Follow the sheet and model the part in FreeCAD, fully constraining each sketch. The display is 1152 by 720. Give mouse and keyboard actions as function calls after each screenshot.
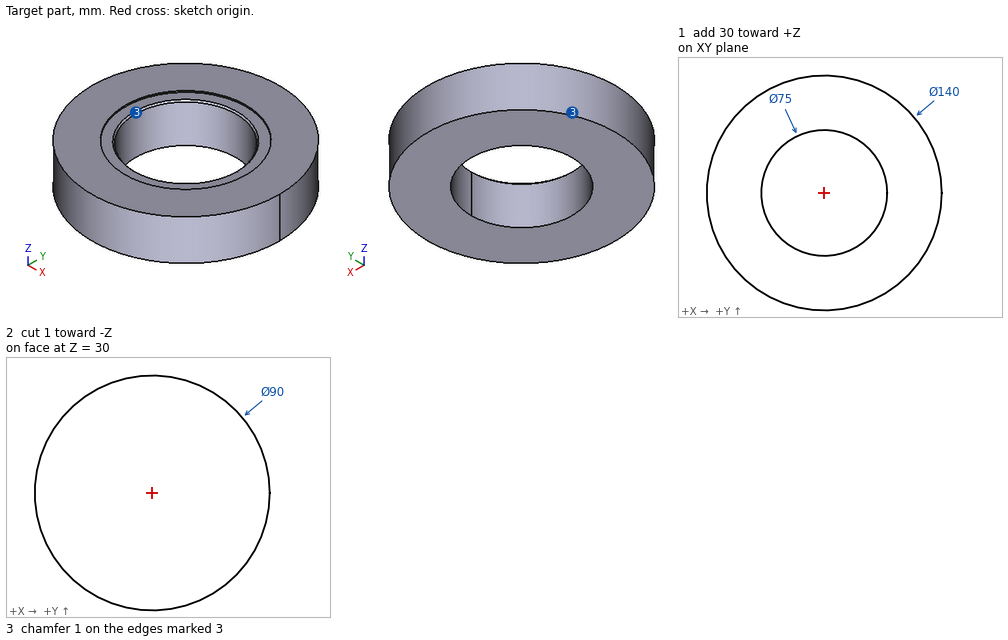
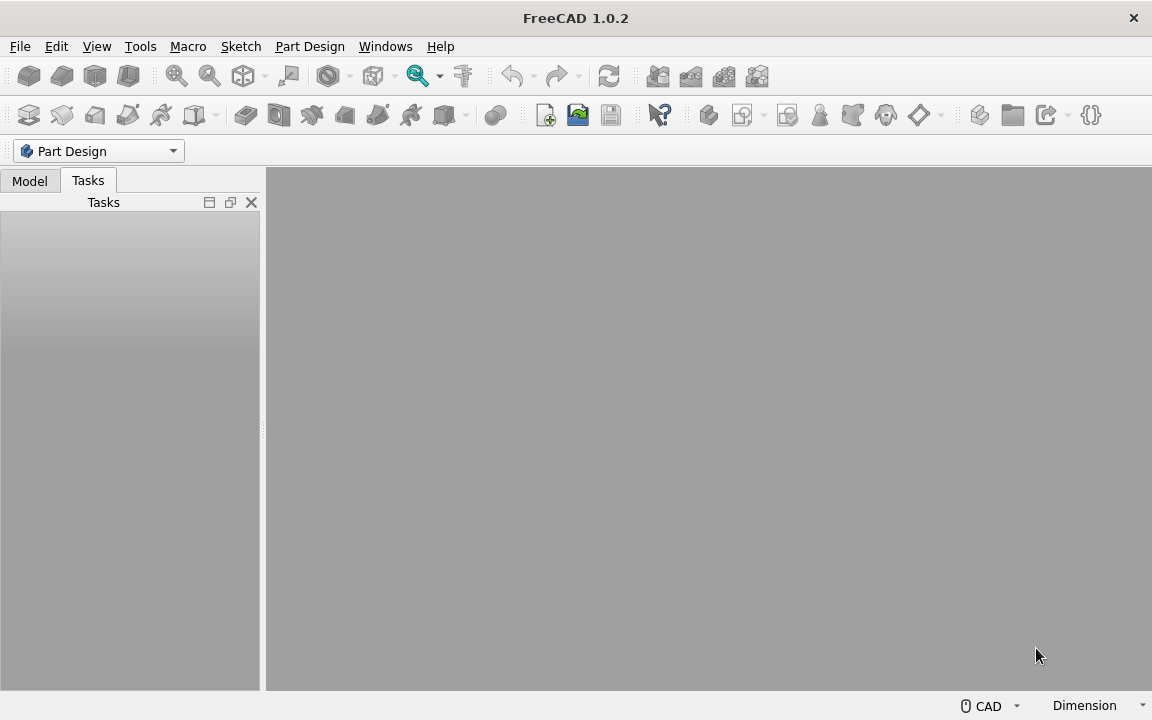
click(545, 116)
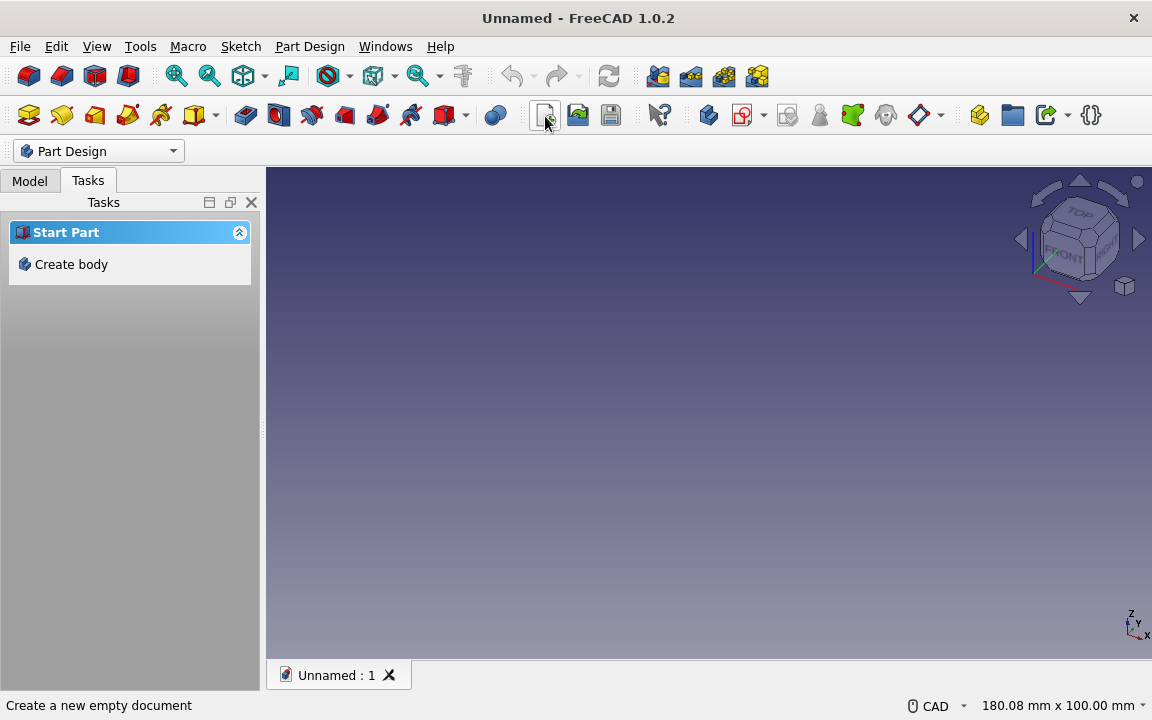
click(742, 116)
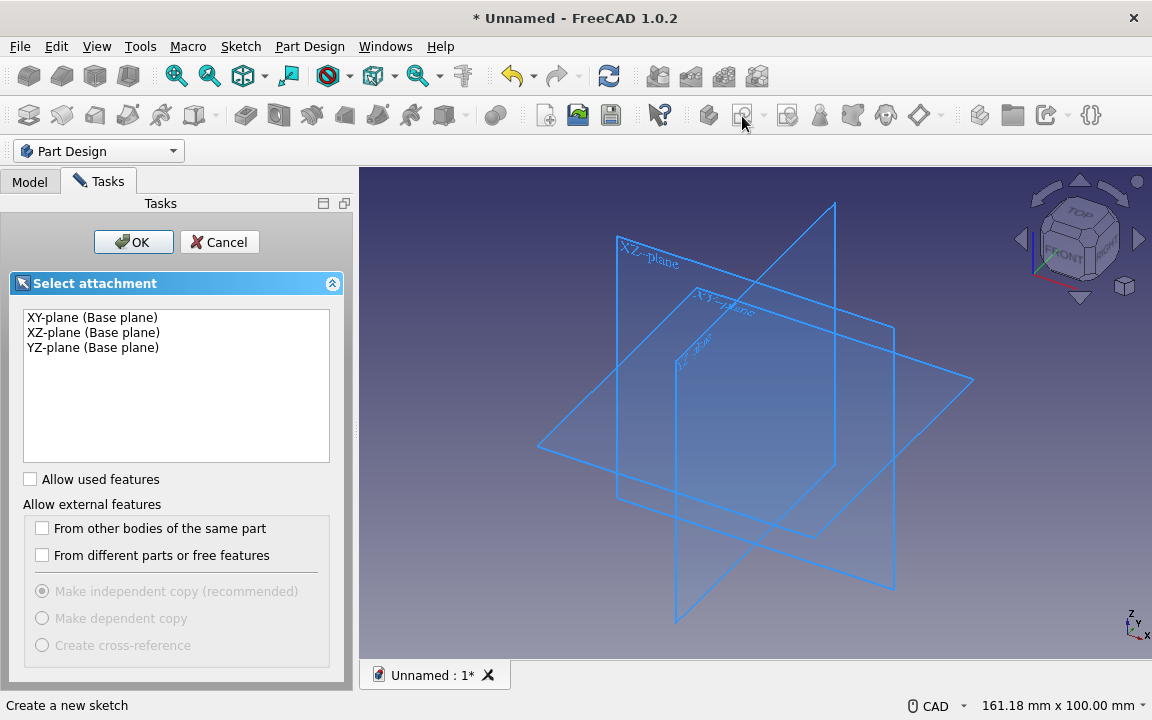
click(84, 318)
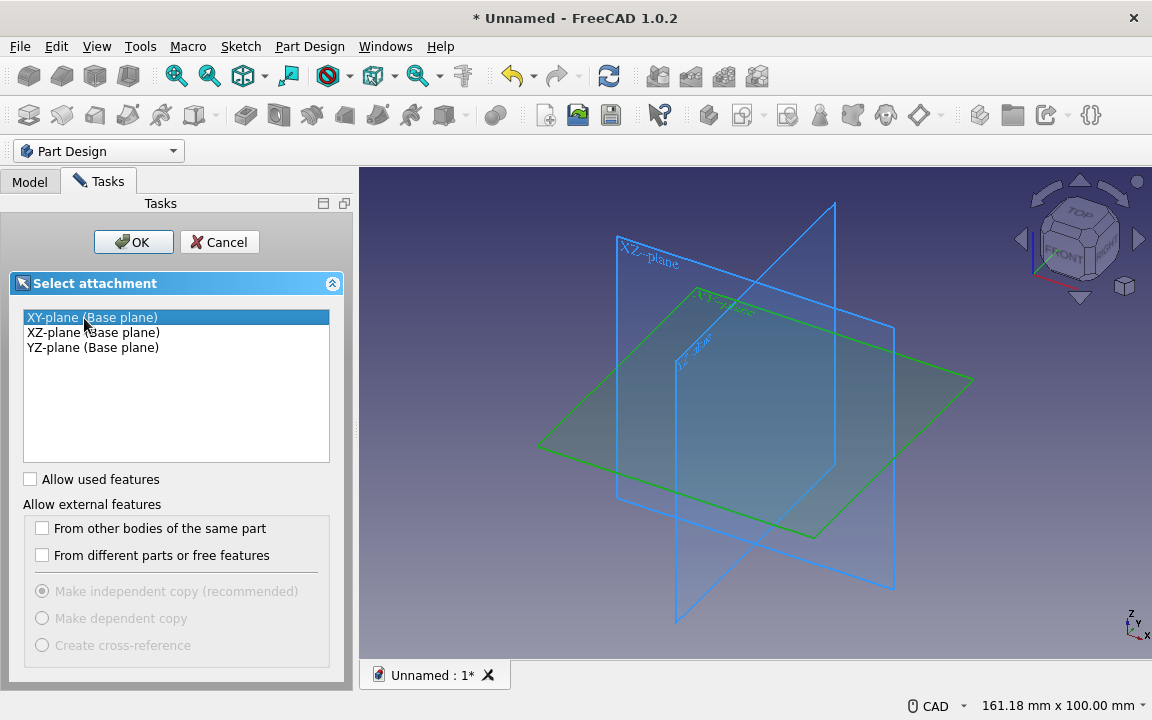
click(134, 242)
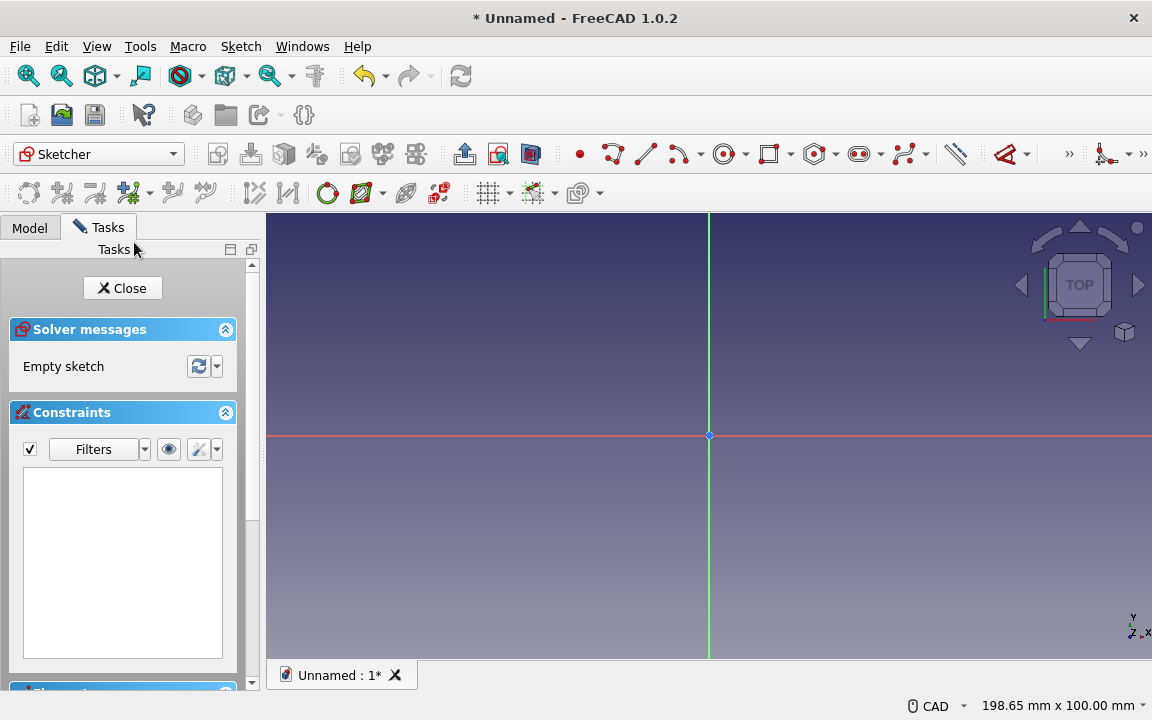
scroll(585, 436, down, 4)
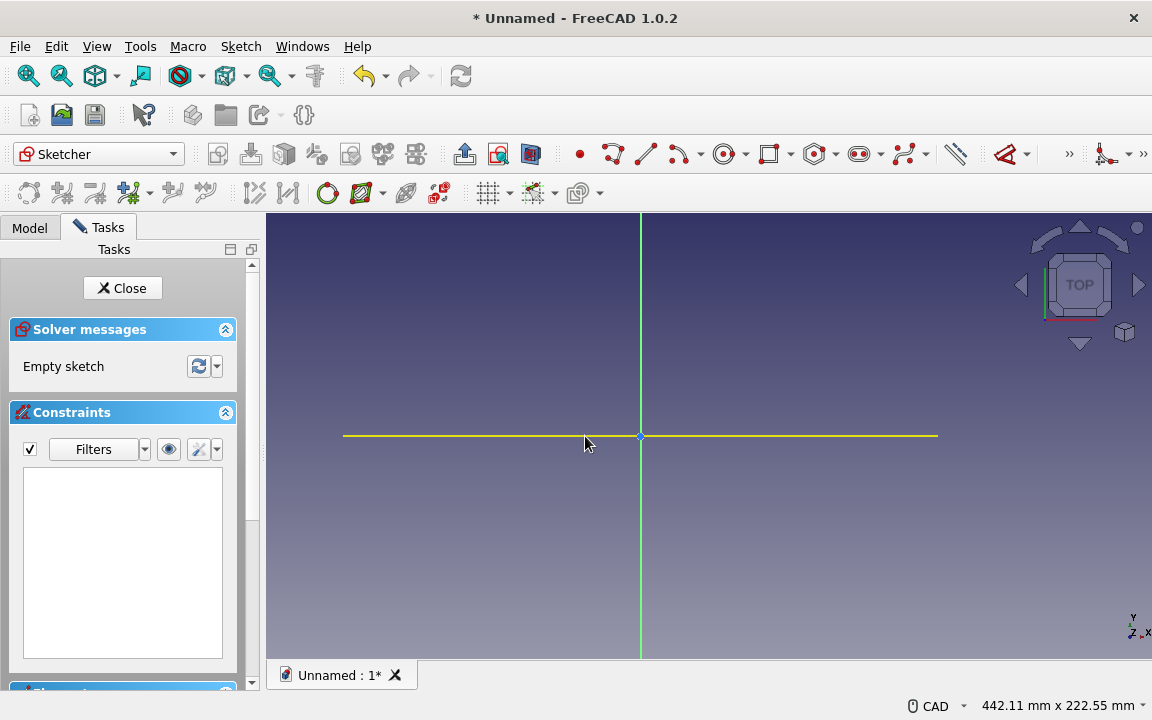
click(724, 154)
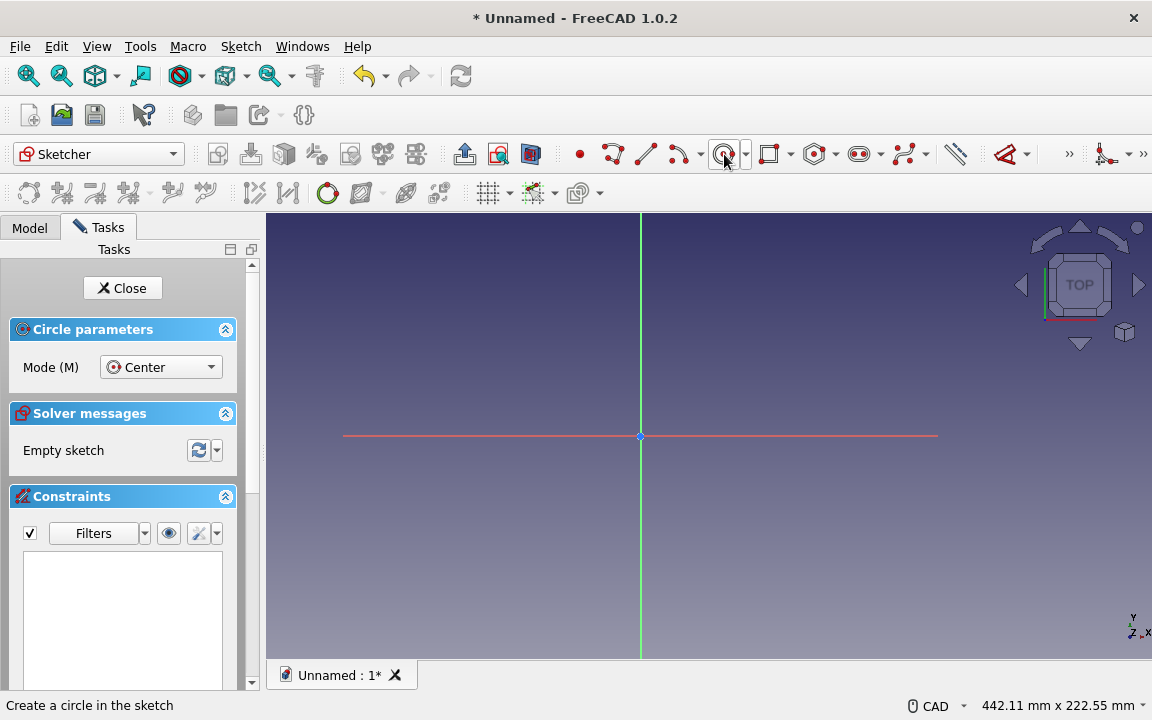
click(641, 436)
move(740, 337)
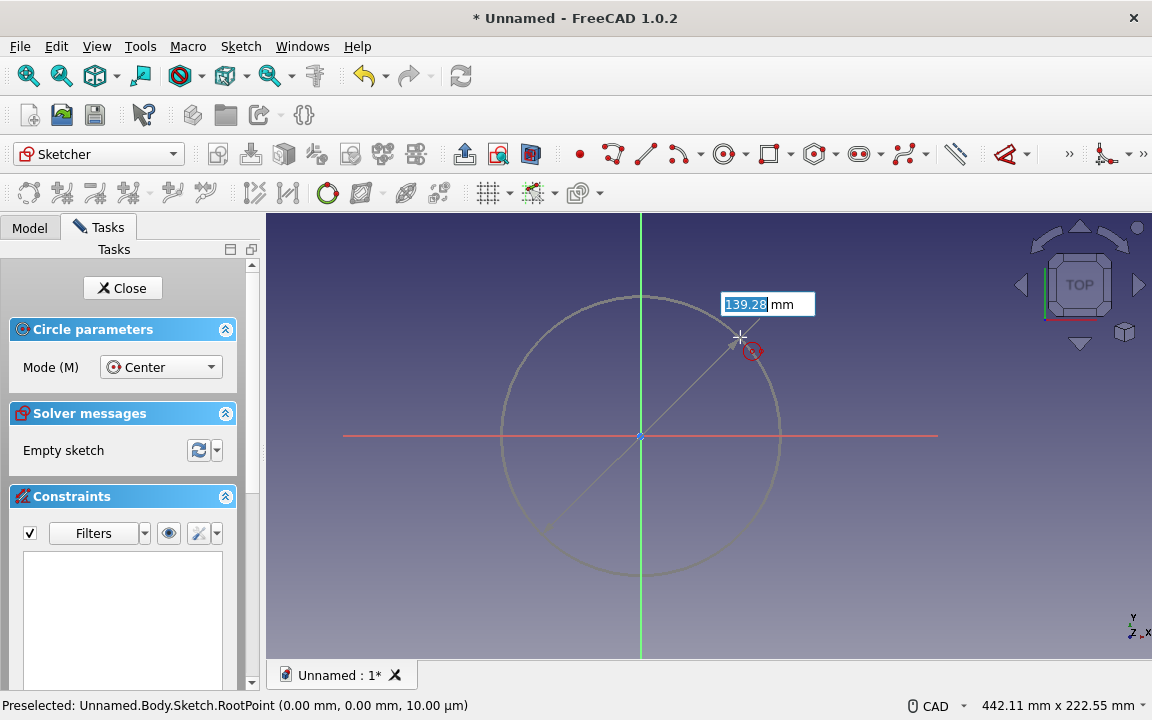
text(140)
key(Return)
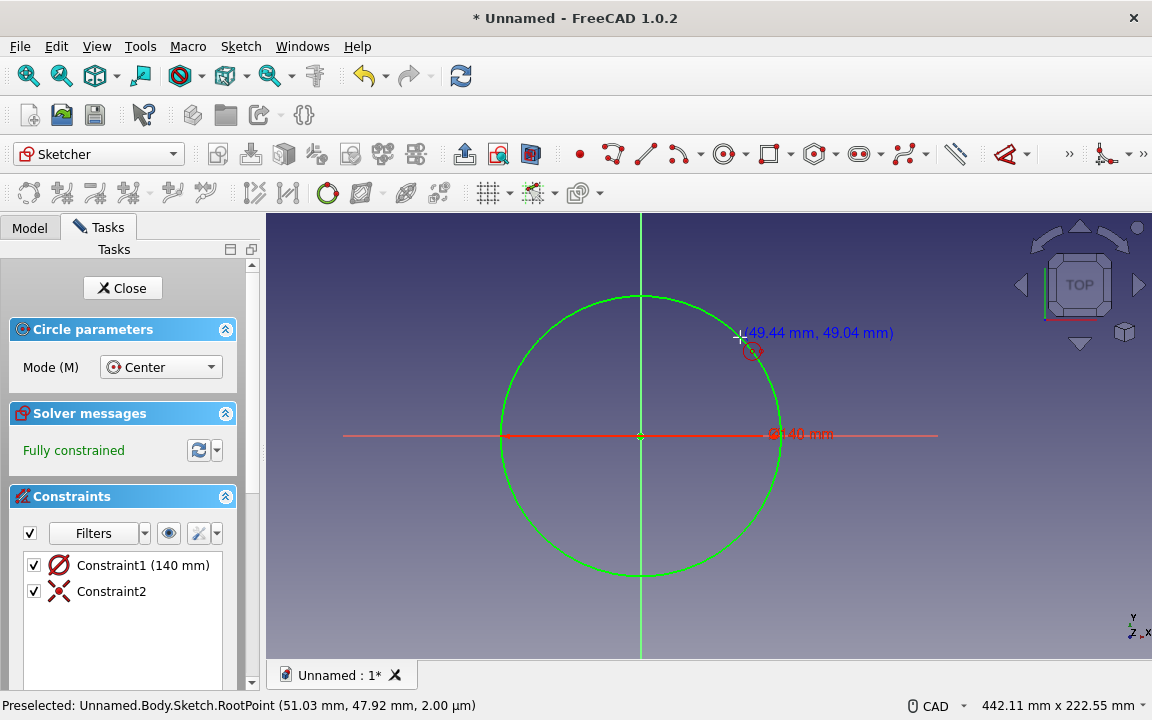
click(641, 436)
move(694, 383)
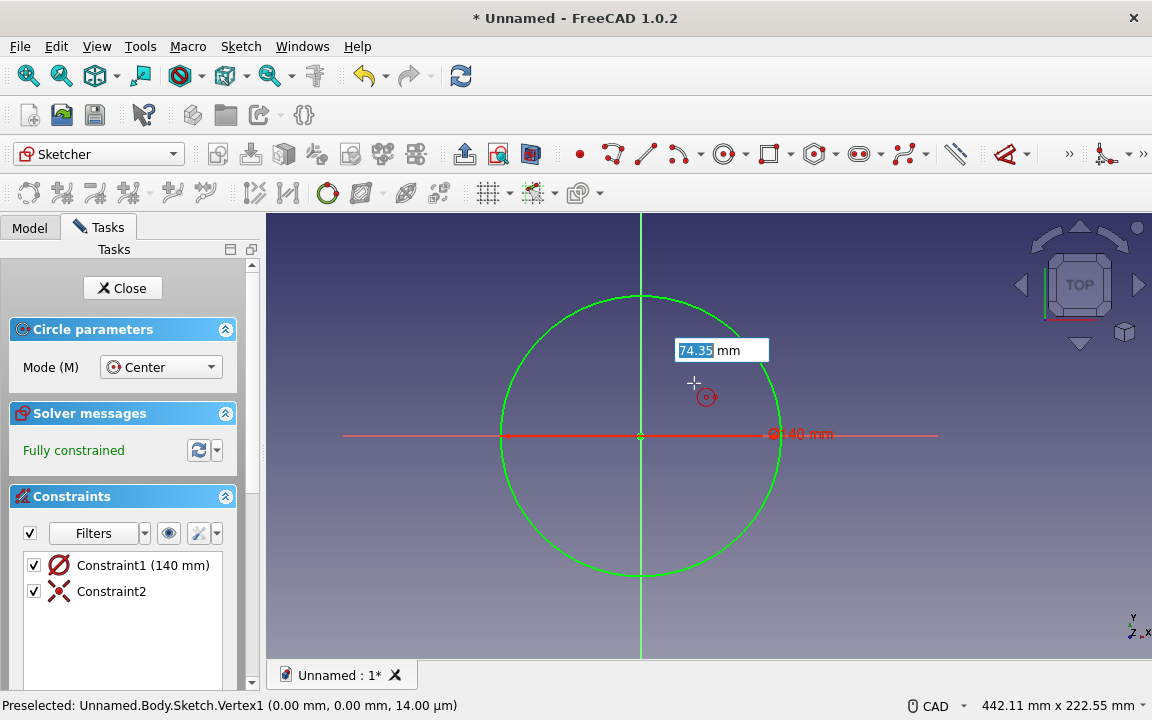
text(75)
key(Return)
key(Escape)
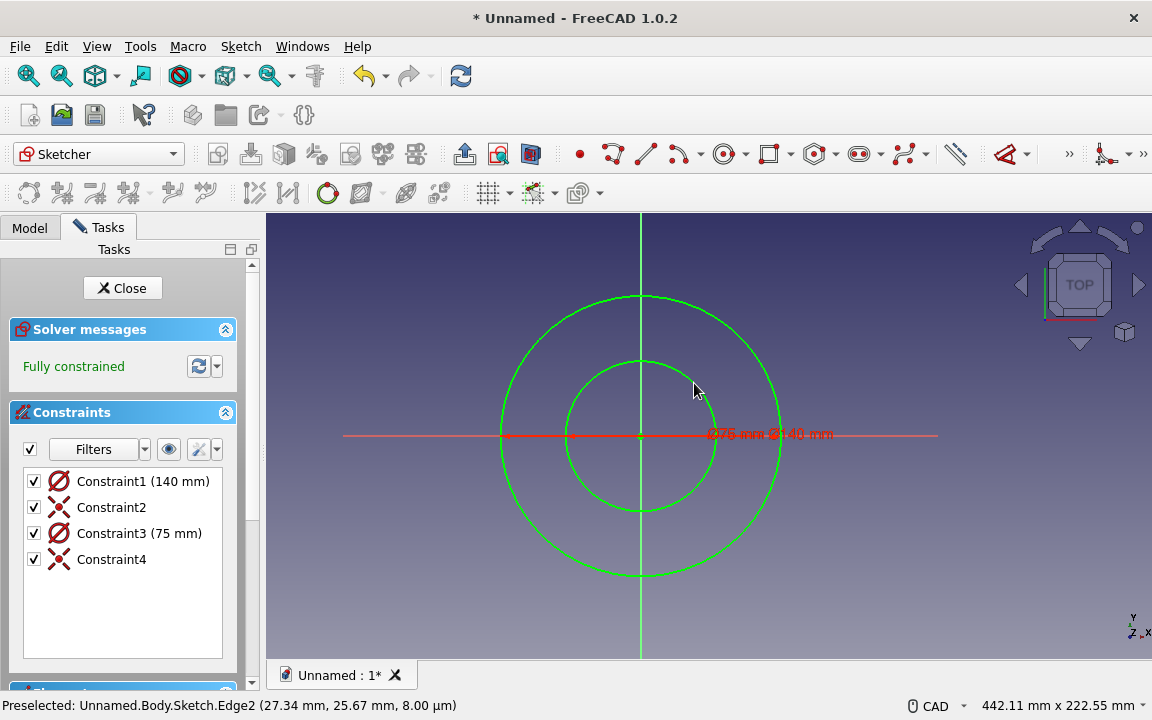
click(123, 288)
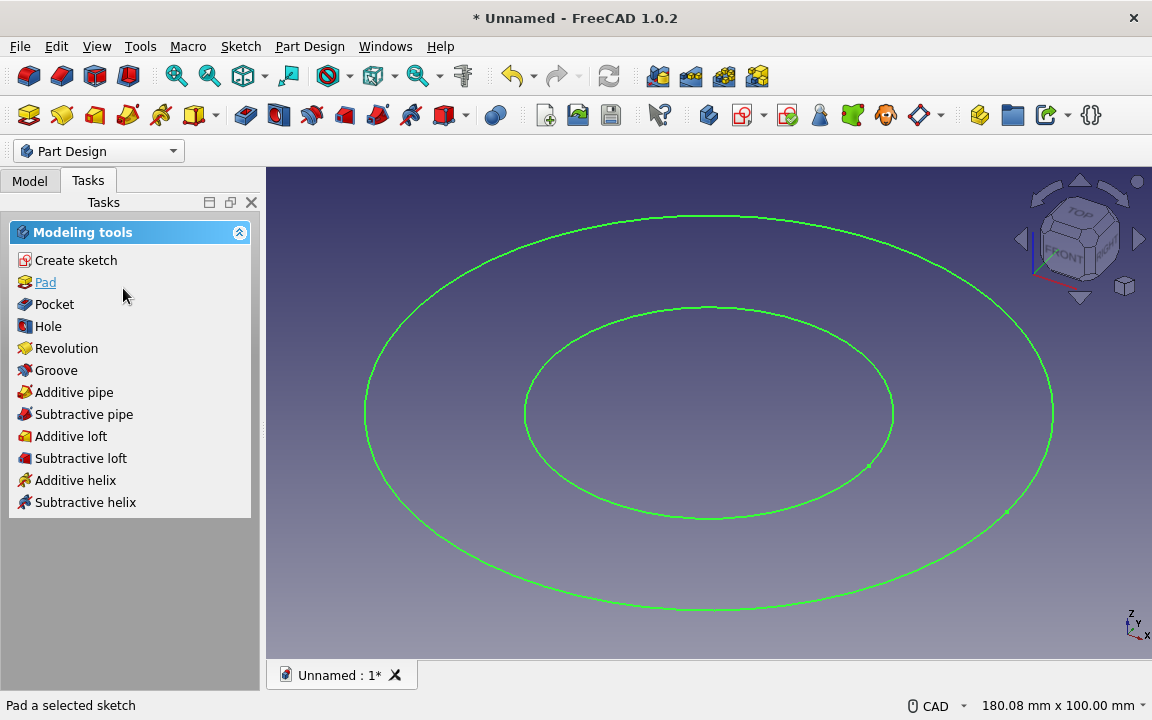
click(29, 116)